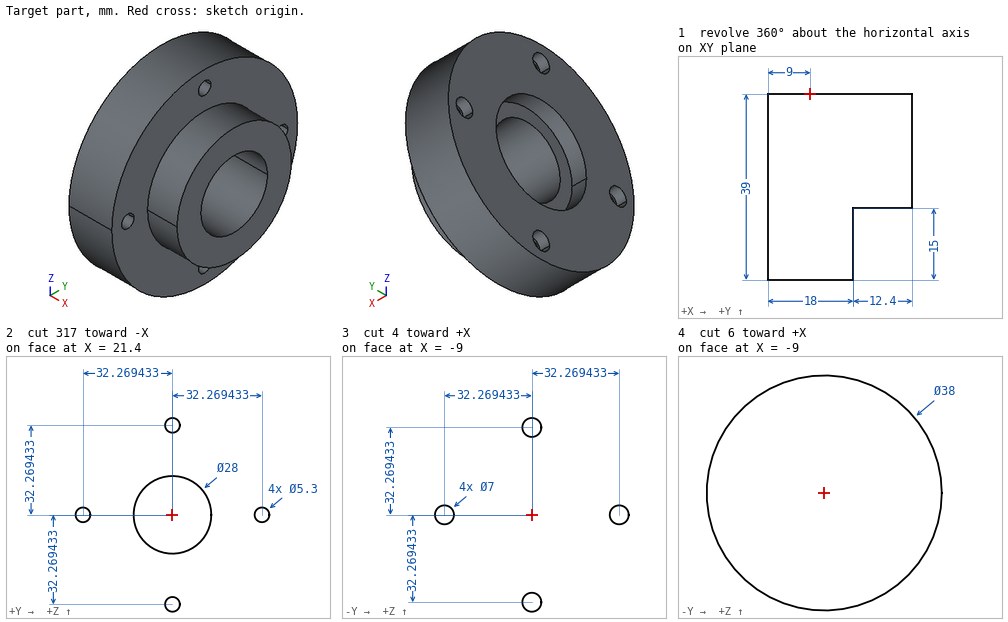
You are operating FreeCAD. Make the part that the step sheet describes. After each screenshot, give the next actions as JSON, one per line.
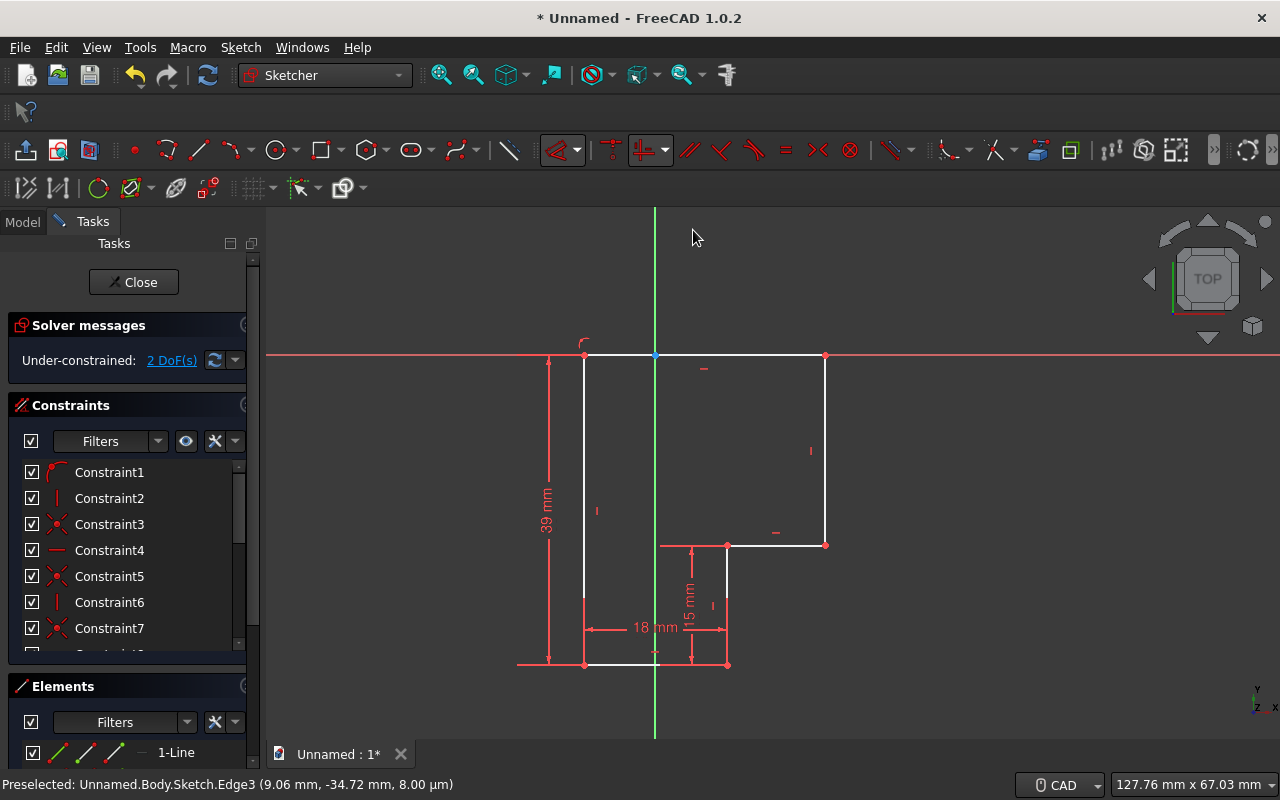
{"action": "left_click", "coordinate": [584, 355]}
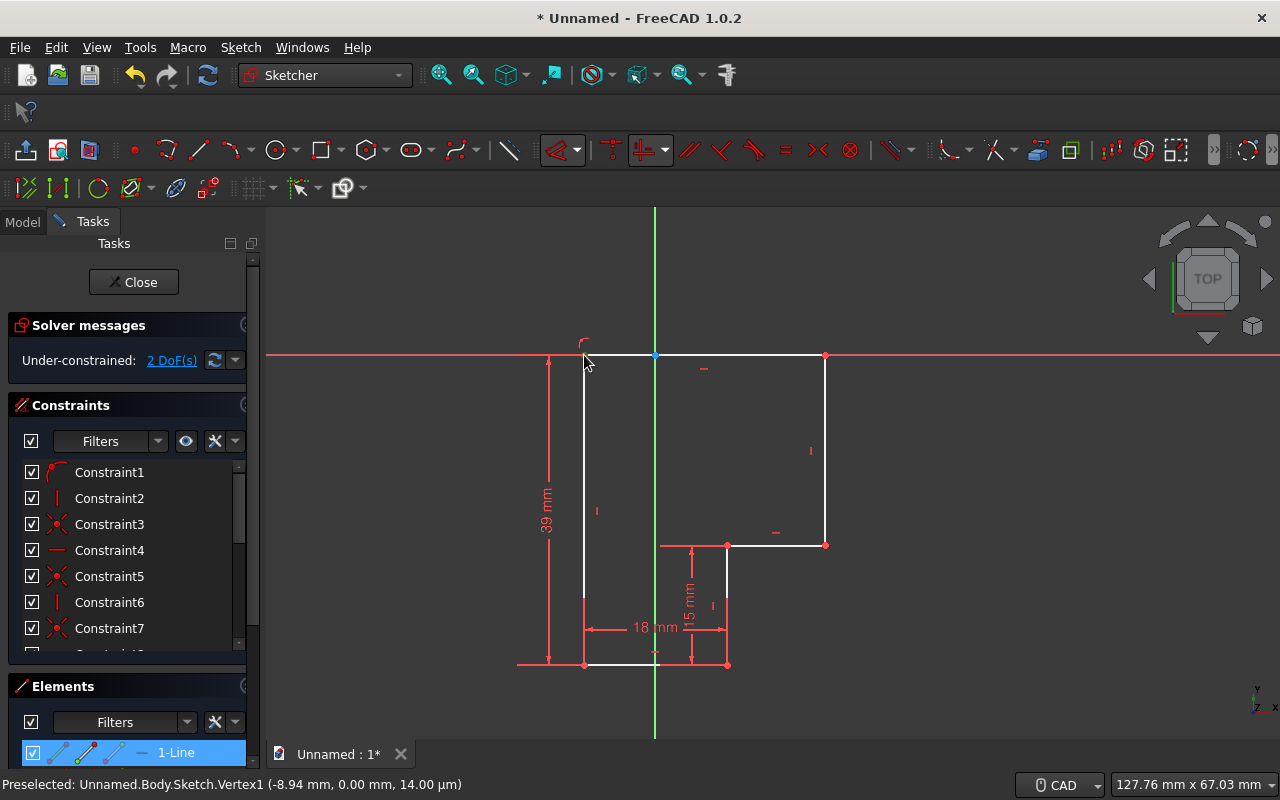
{"action": "left_click", "coordinate": [580, 150]}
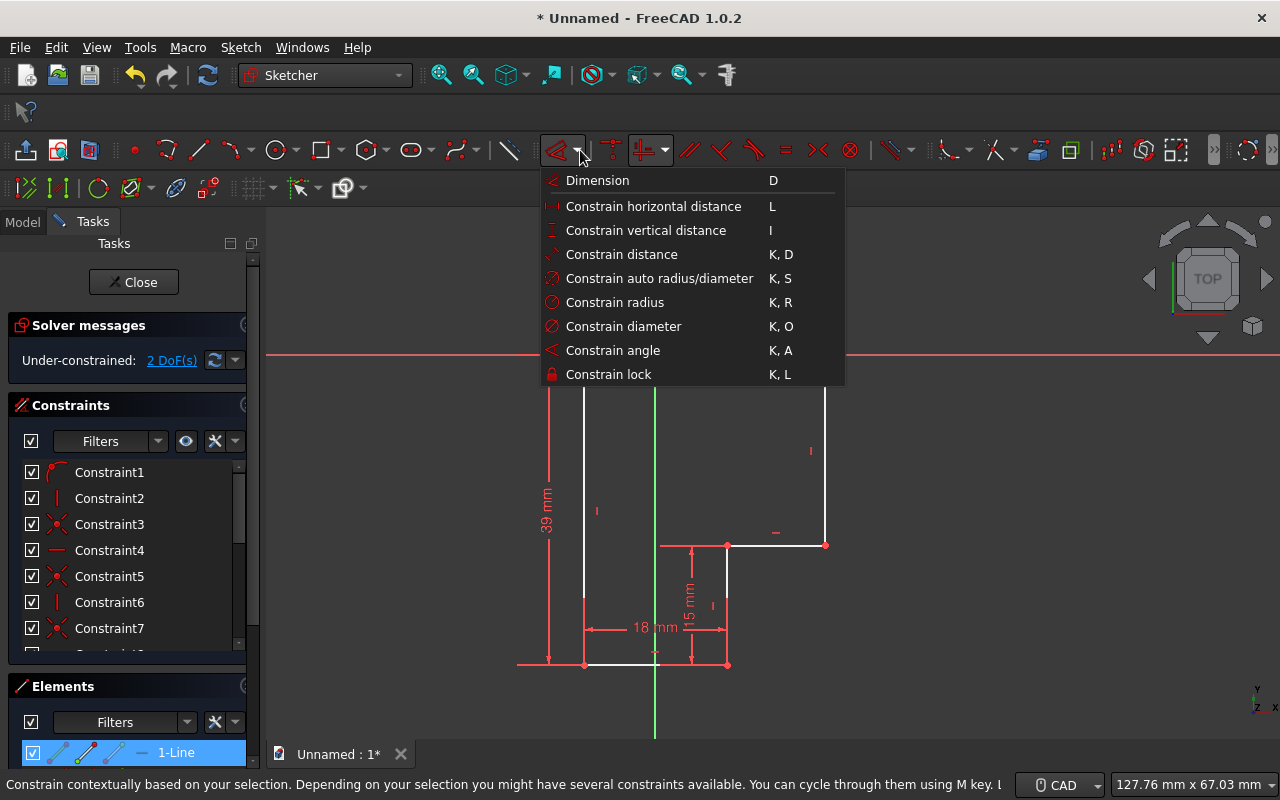
{"action": "left_click", "coordinate": [693, 206]}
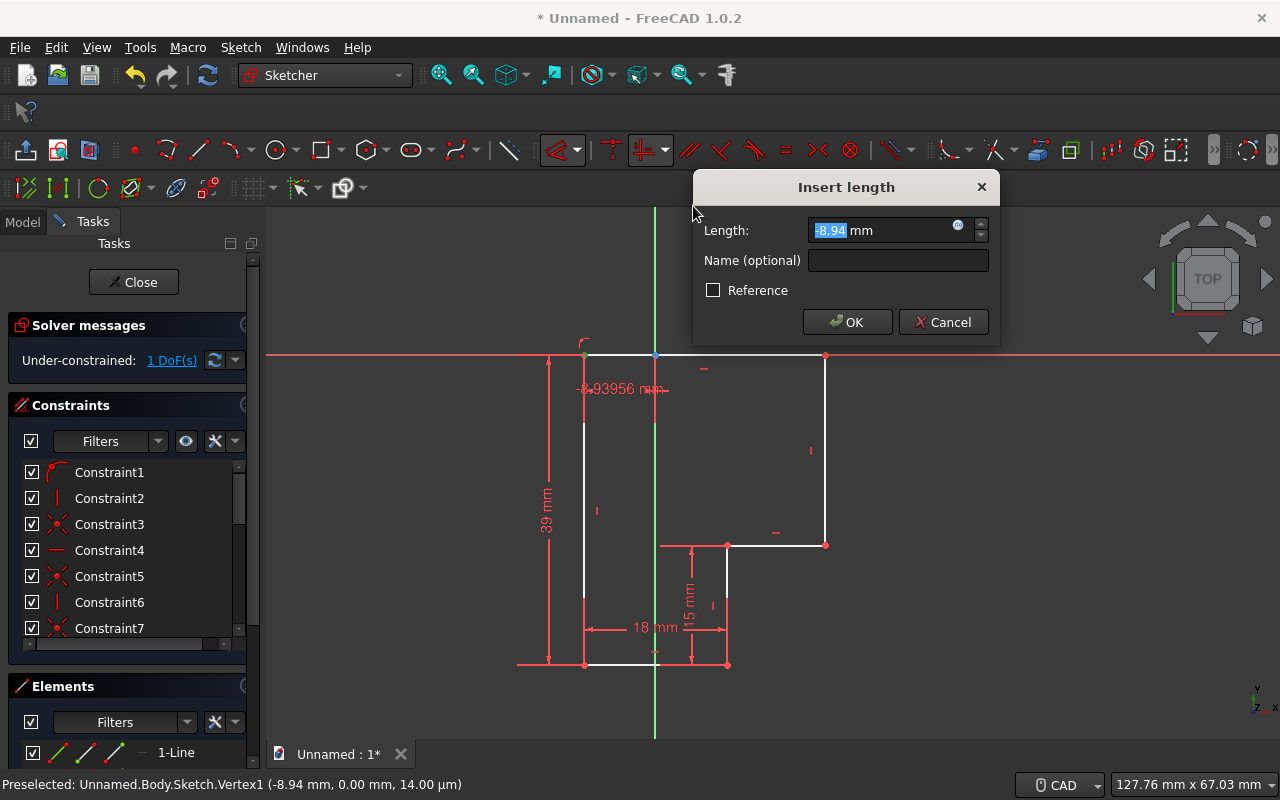
{"action": "type", "text": "-9"}
{"action": "key", "text": "Return"}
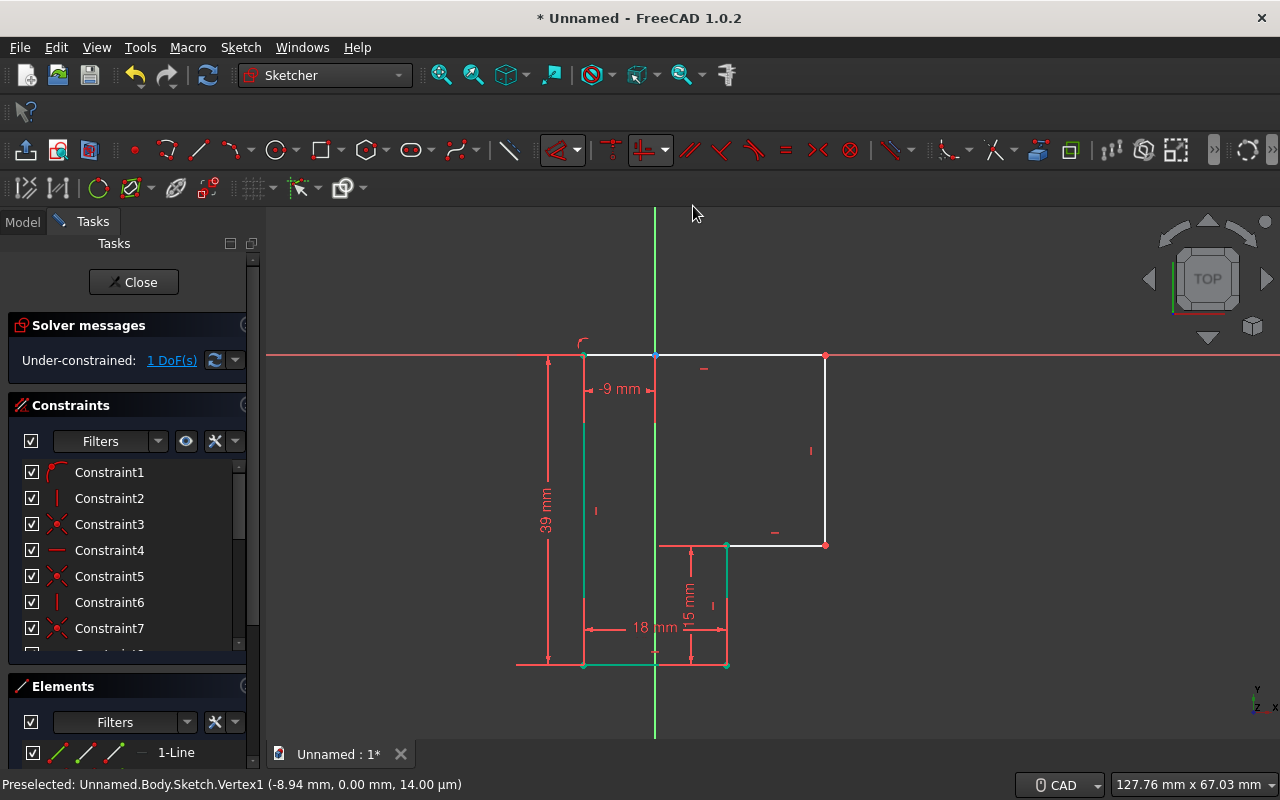
{"action": "left_click", "coordinate": [756, 546]}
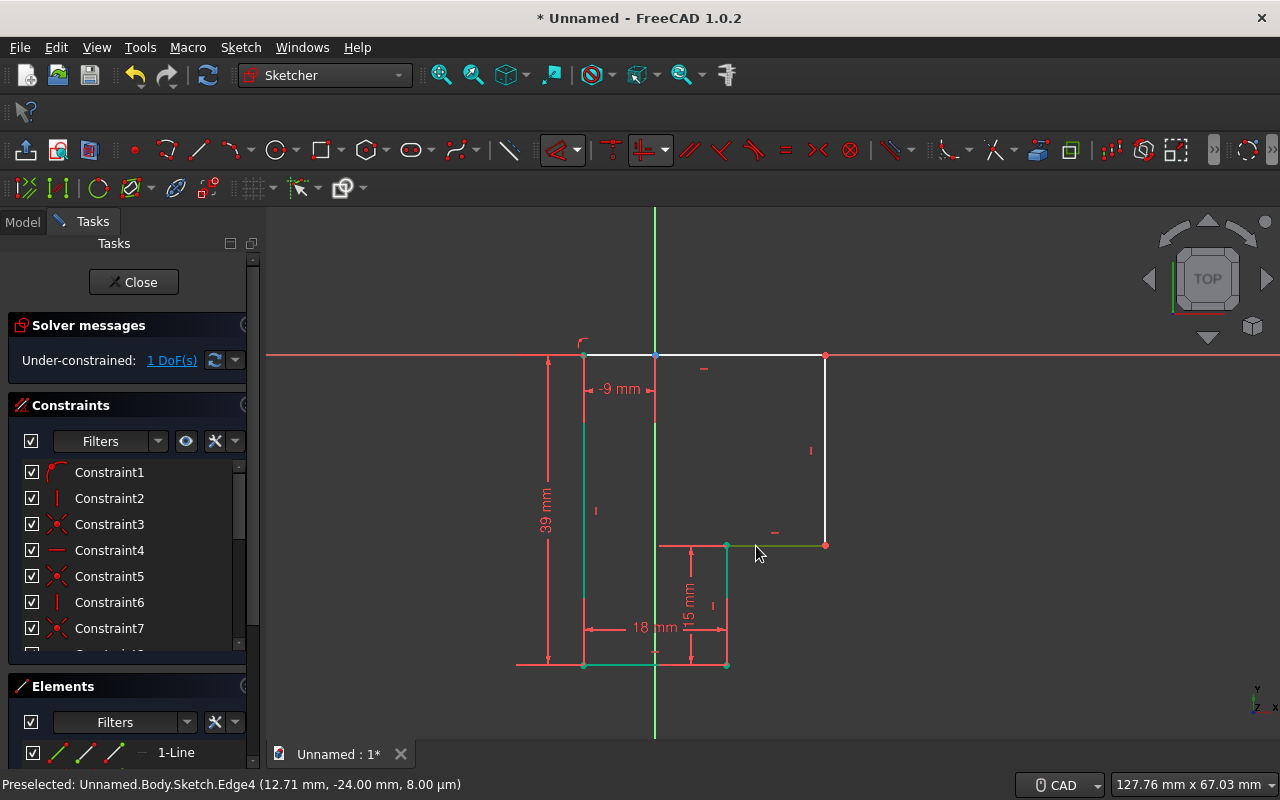
{"action": "left_click", "coordinate": [580, 150]}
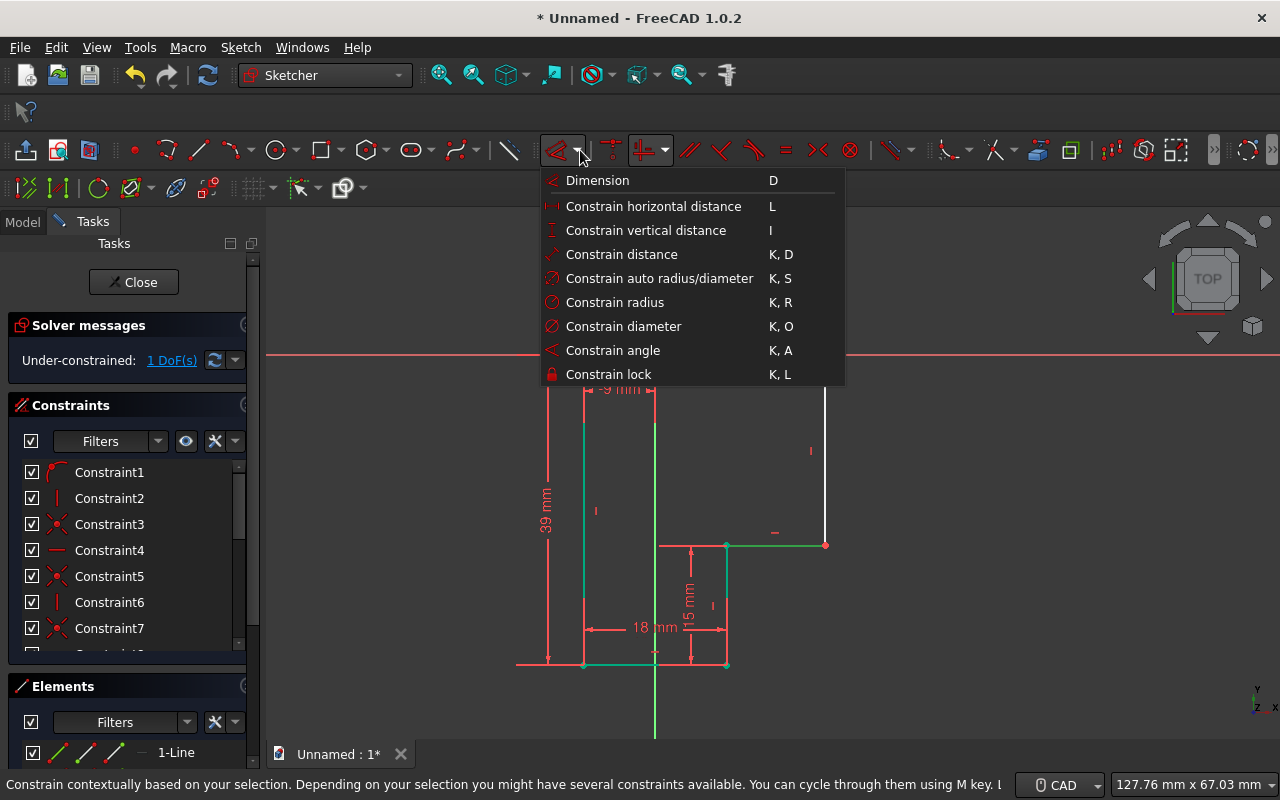
{"action": "left_click", "coordinate": [693, 206]}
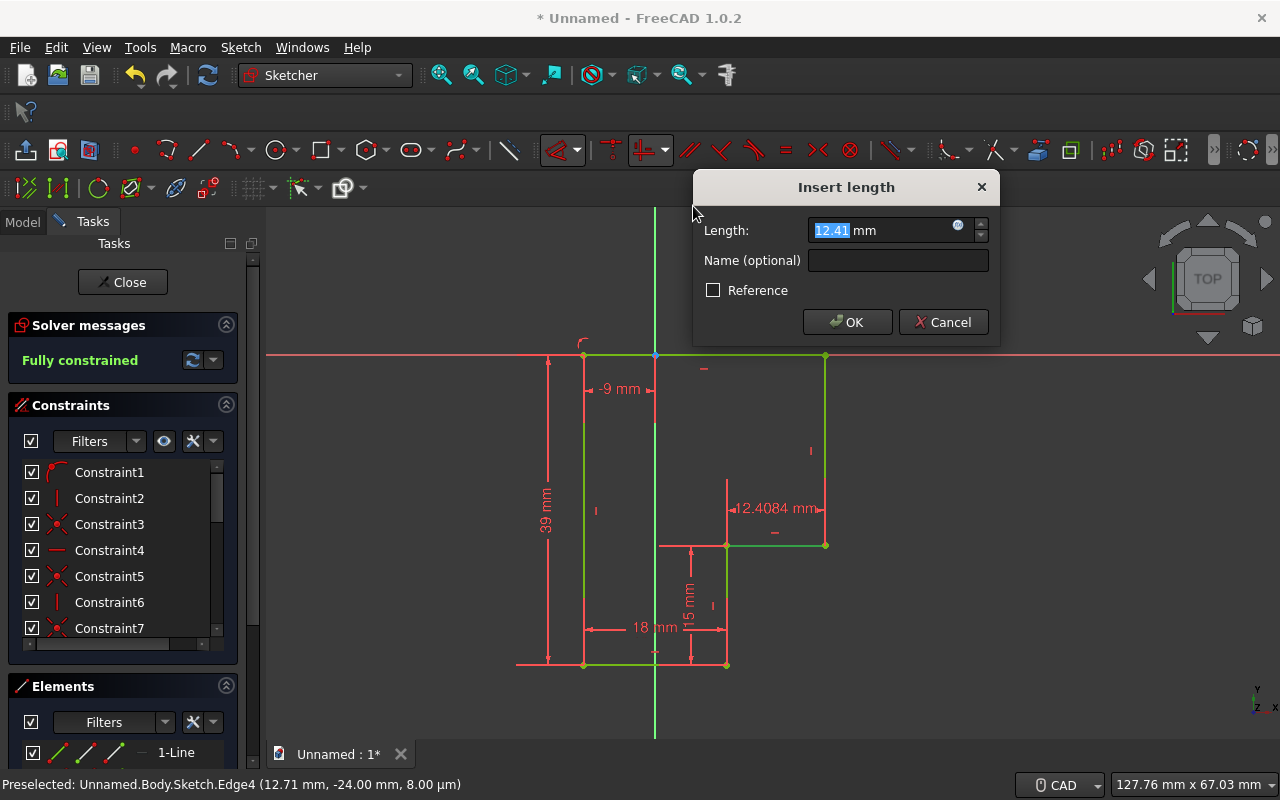
{"action": "type", "text": "12.4"}
{"action": "key", "text": "Return"}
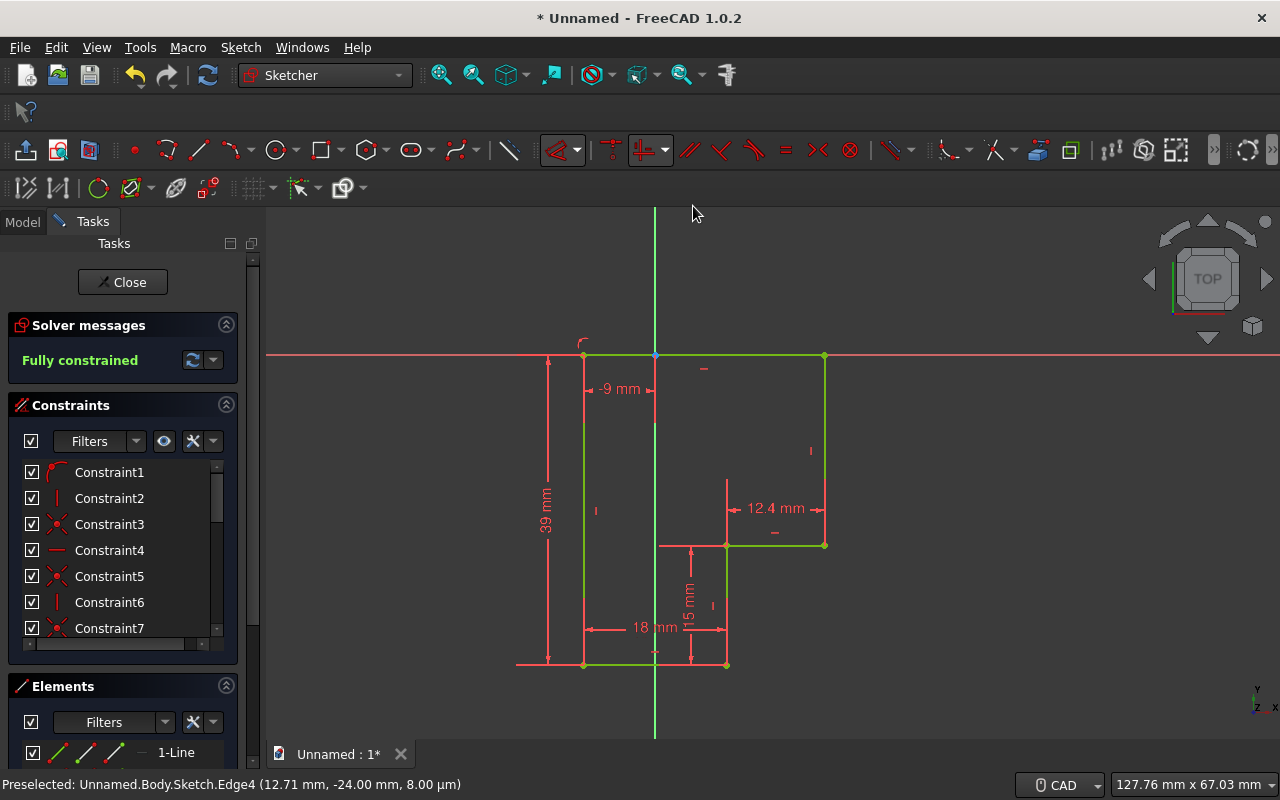
{"action": "left_click", "coordinate": [123, 282]}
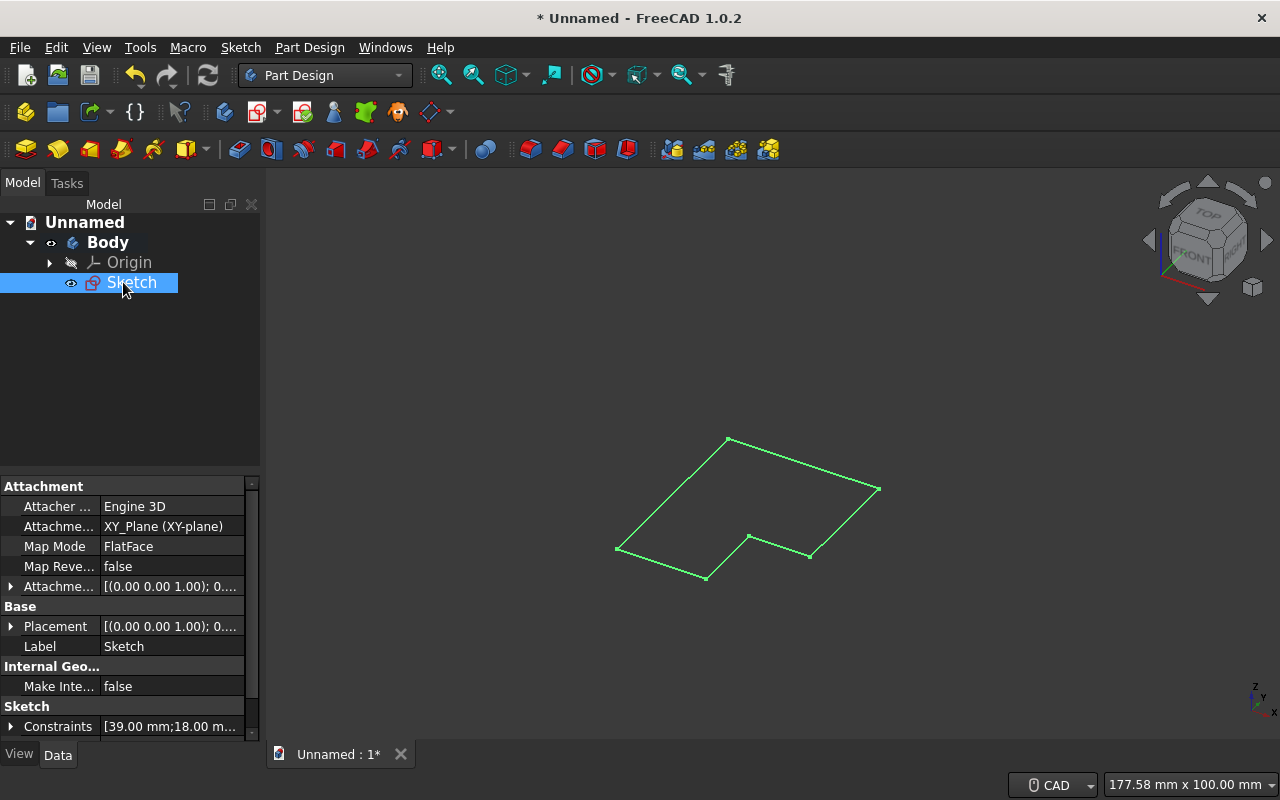
{"action": "left_click", "coordinate": [58, 150]}